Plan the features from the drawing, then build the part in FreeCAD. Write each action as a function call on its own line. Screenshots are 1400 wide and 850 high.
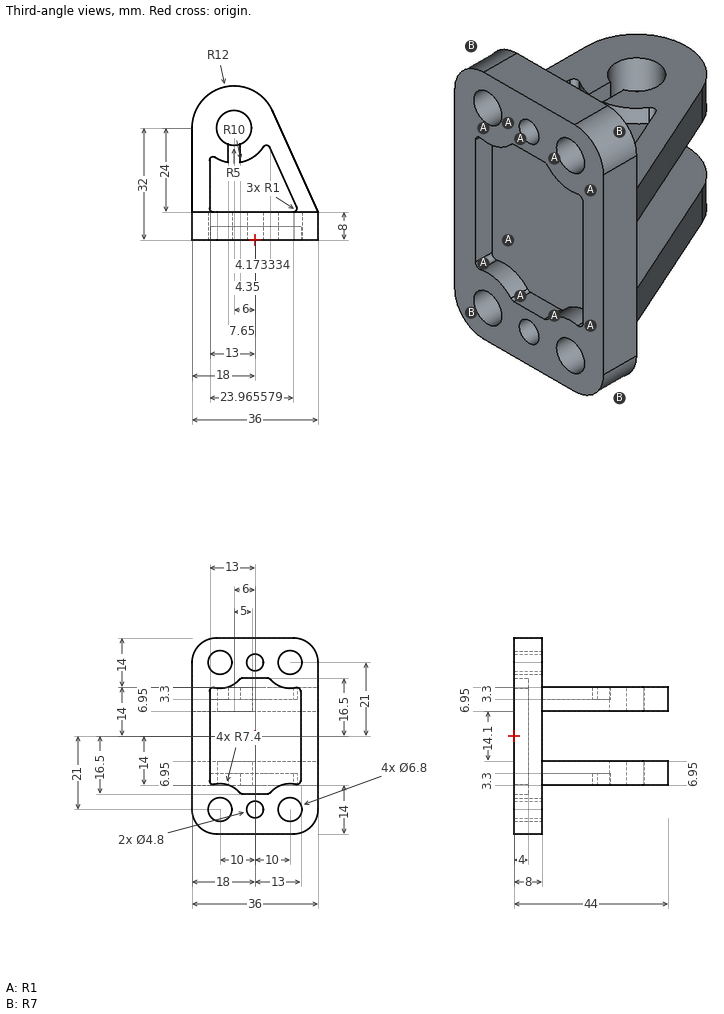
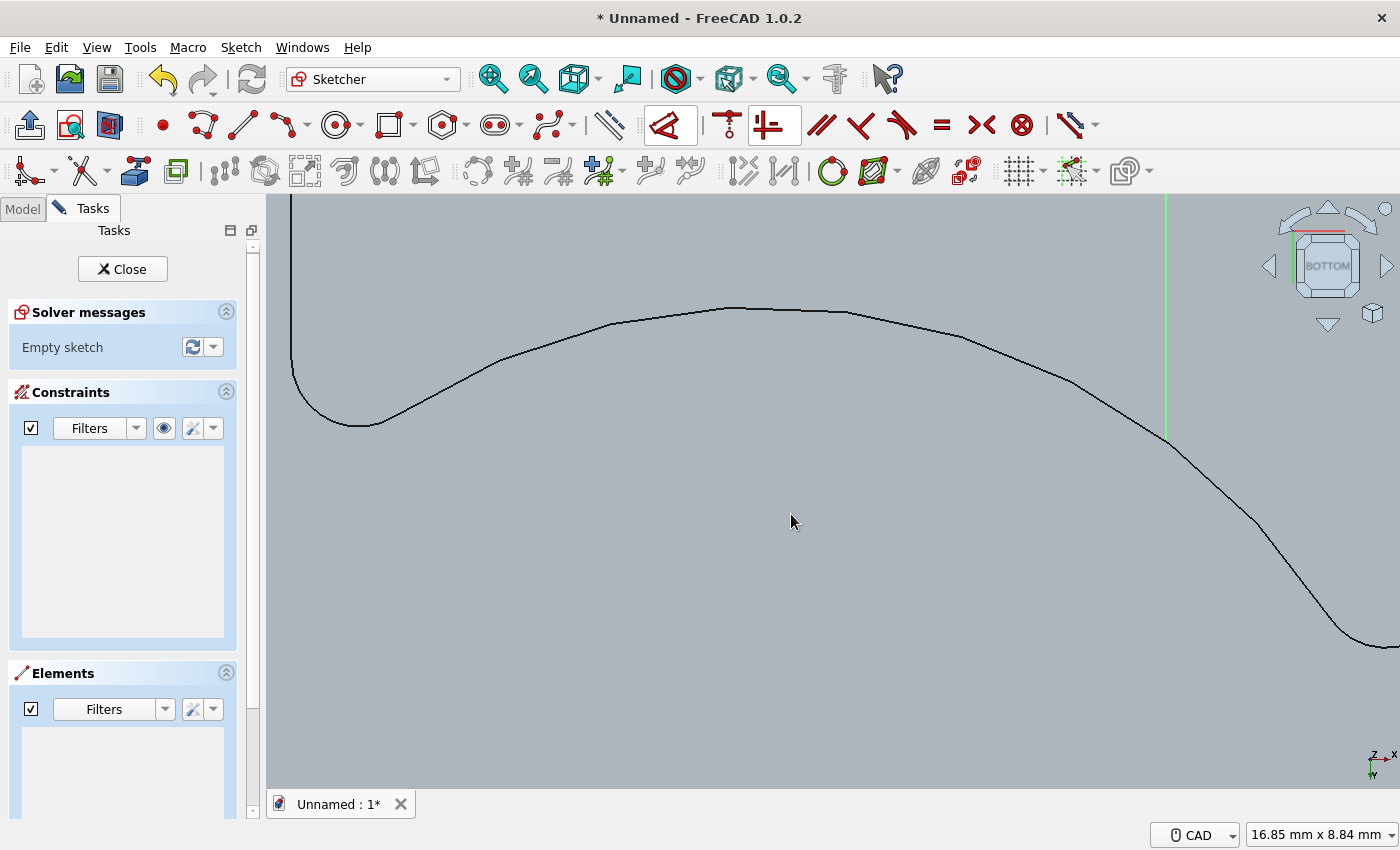
click(244, 126)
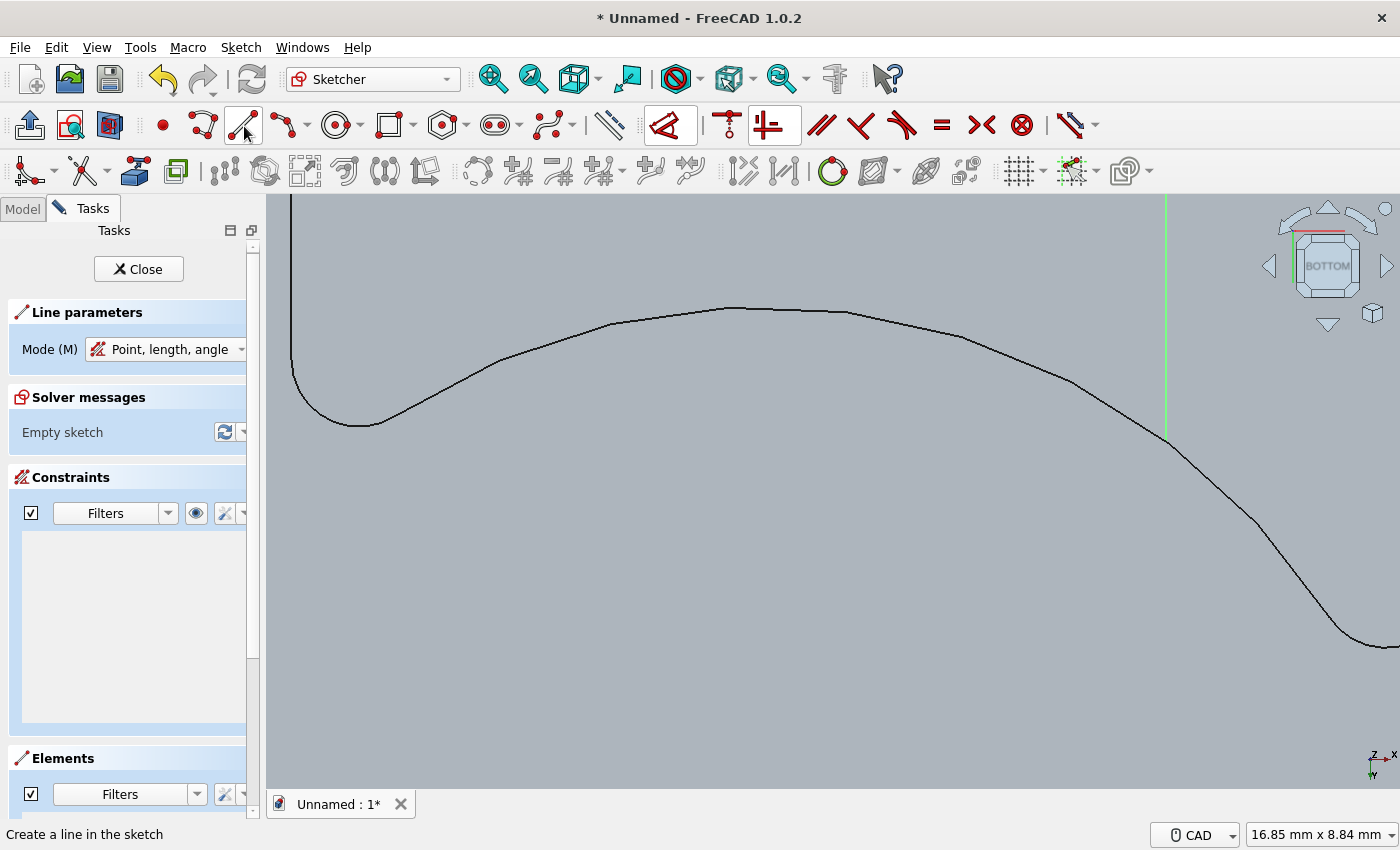
click(652, 316)
click(652, 662)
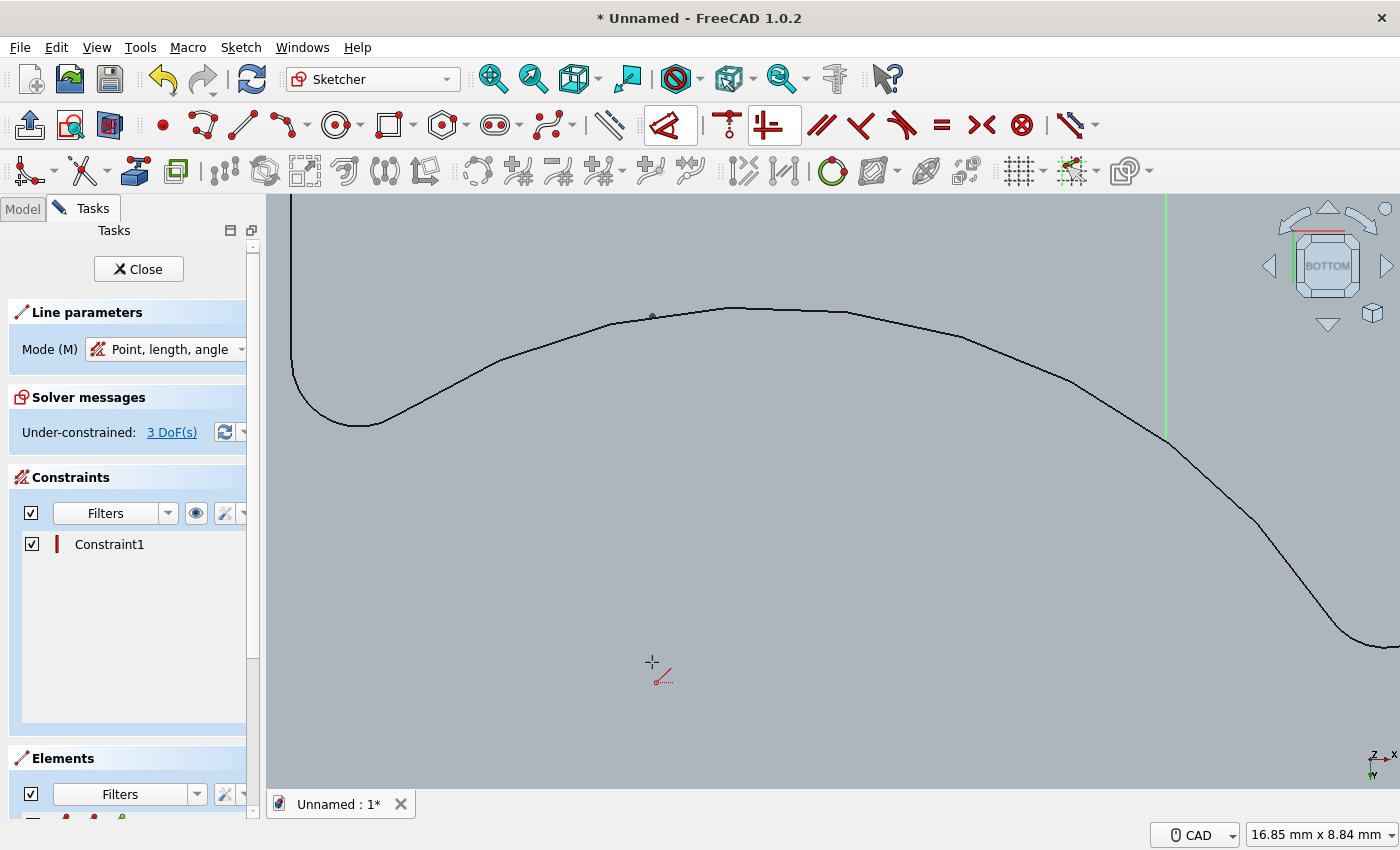
click(874, 662)
click(874, 316)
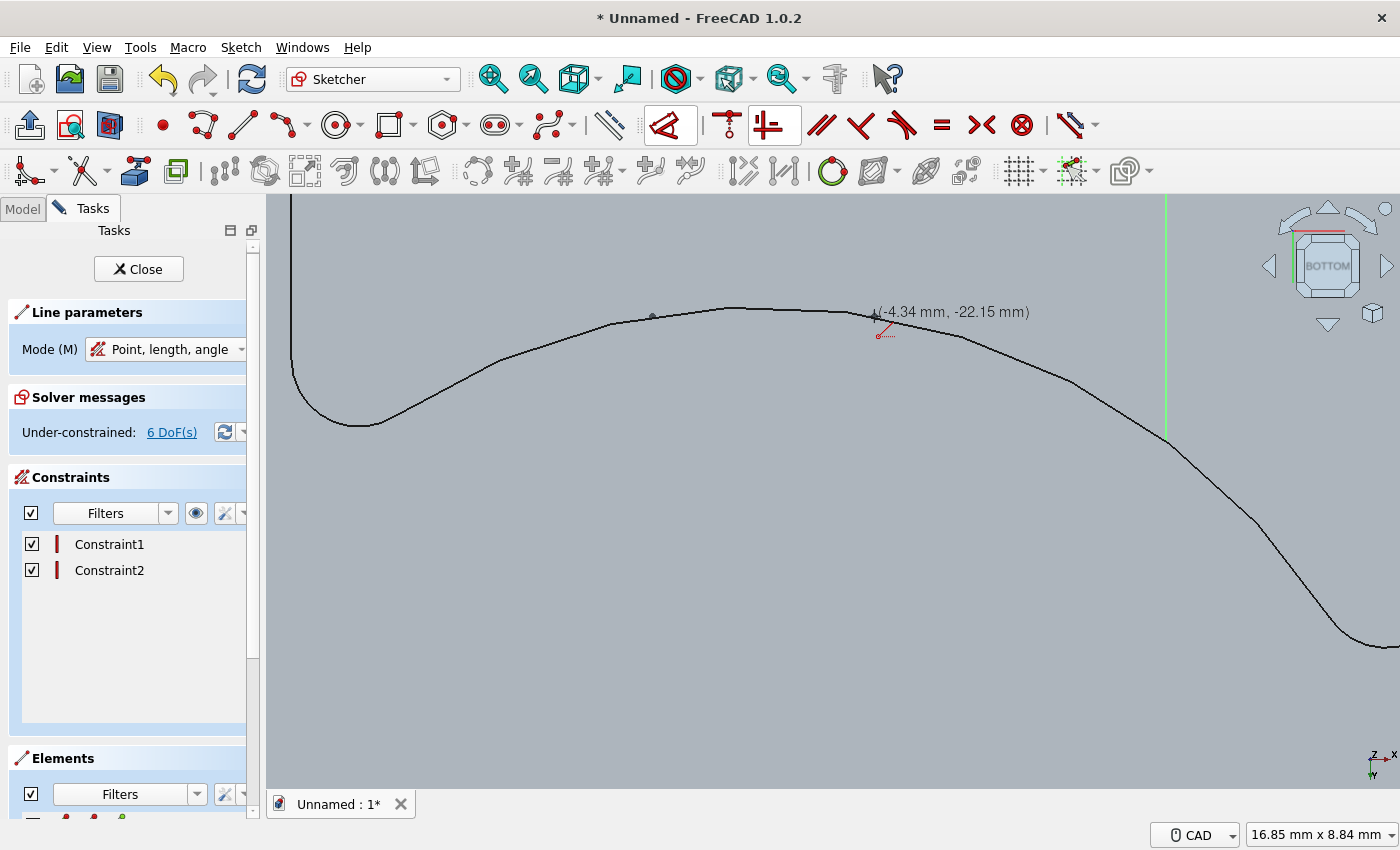
key(g)
key(3)
key(a)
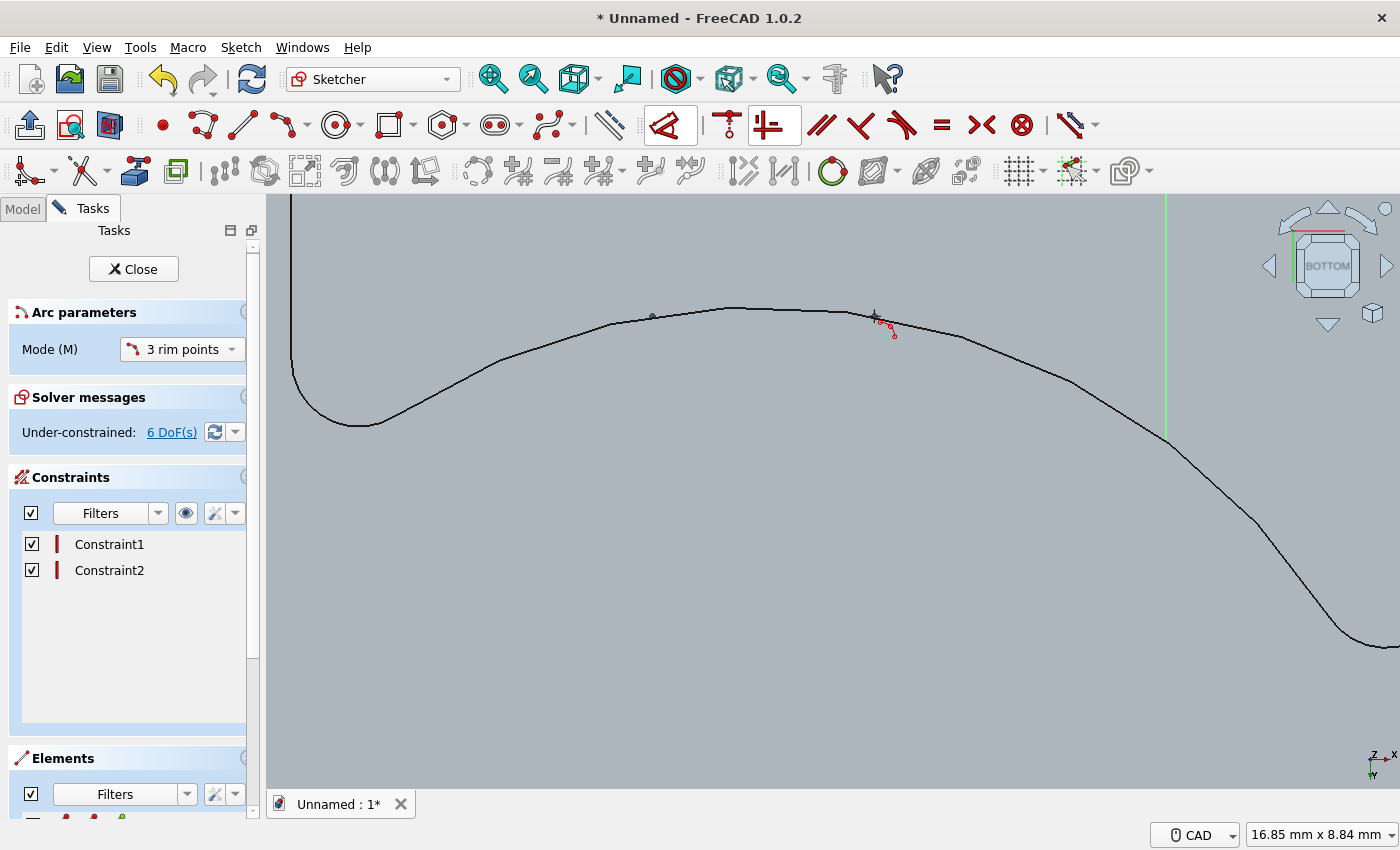
click(652, 663)
click(874, 663)
click(763, 643)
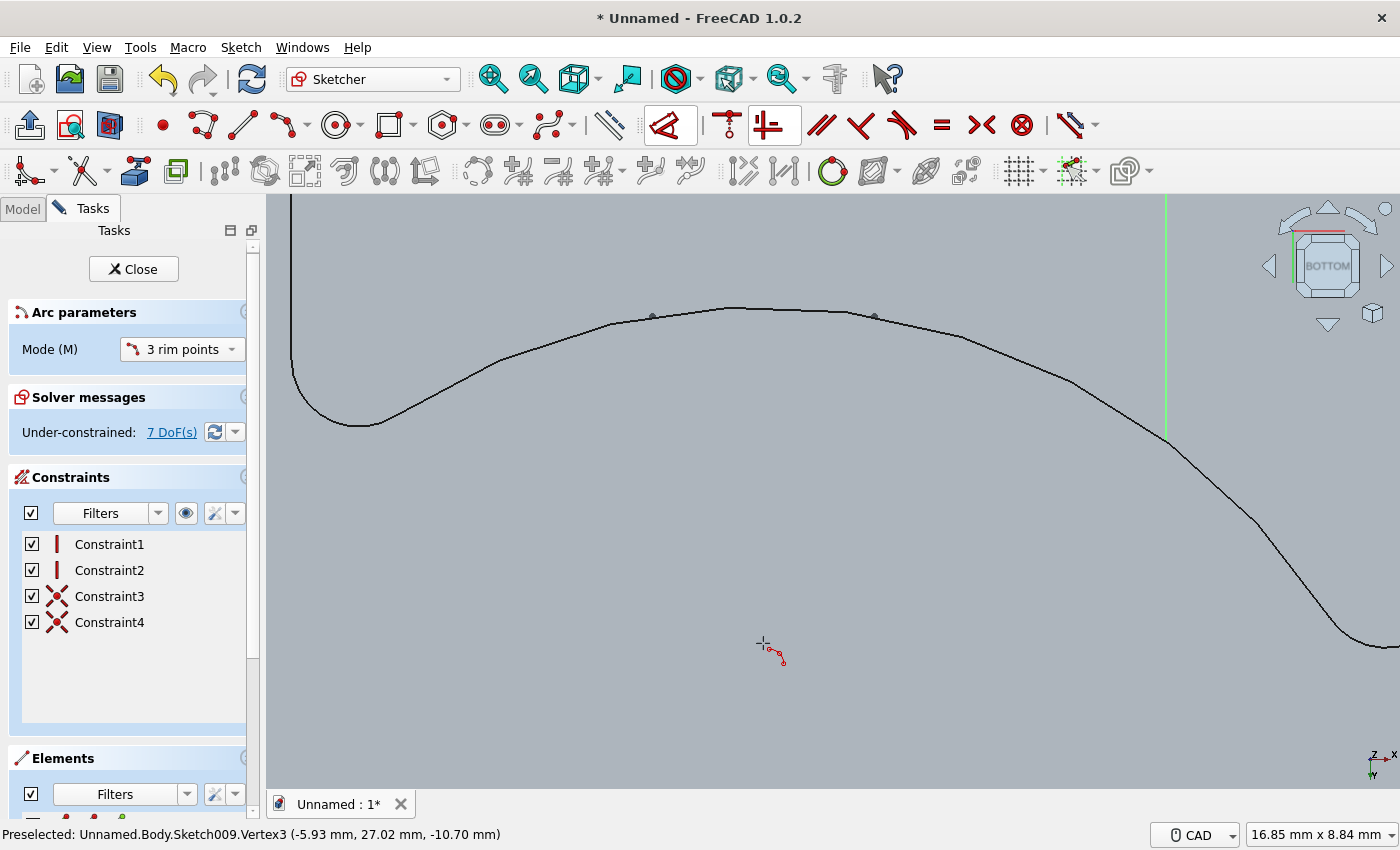
click(874, 317)
click(652, 317)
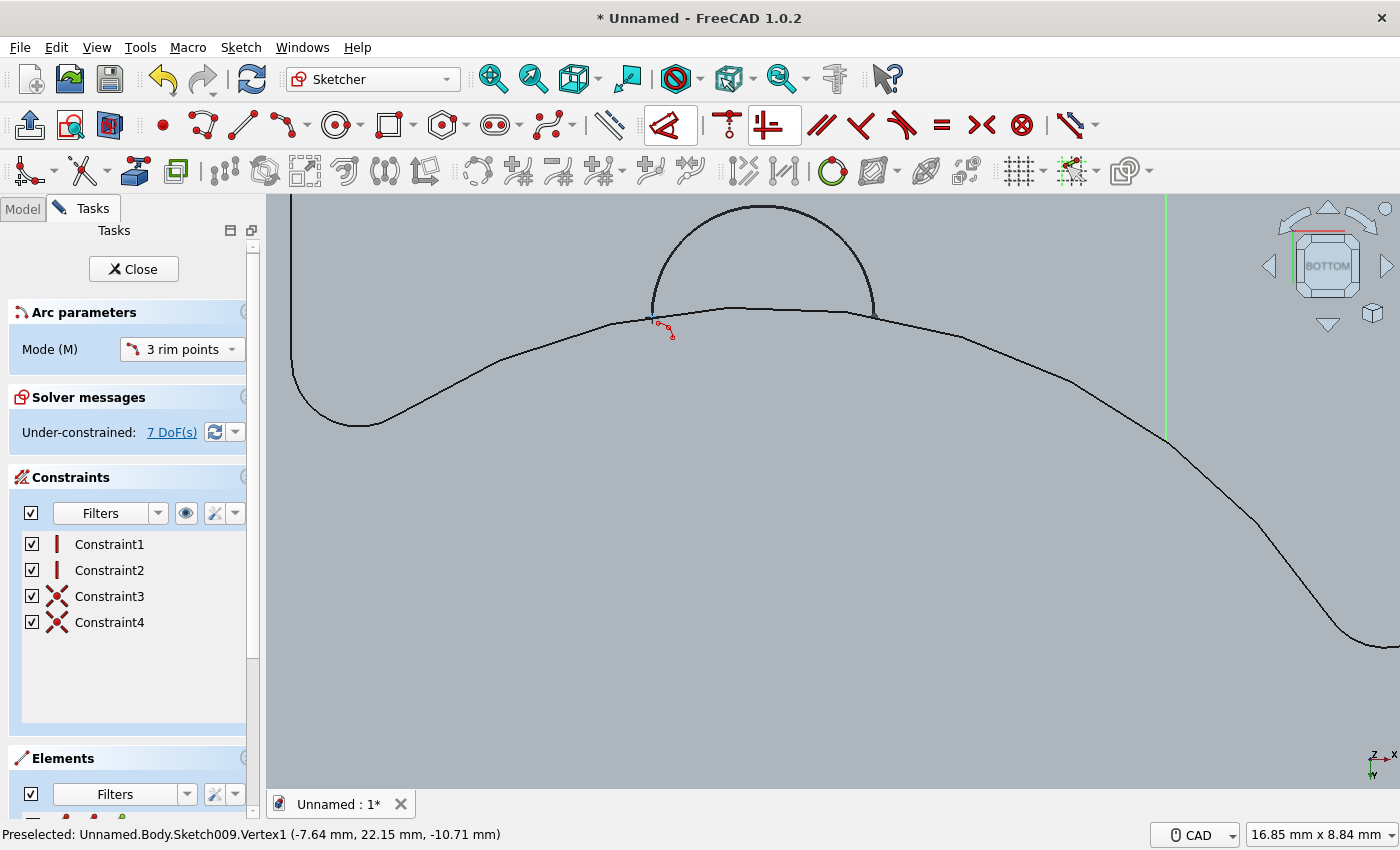
scroll(763, 307, up, 3)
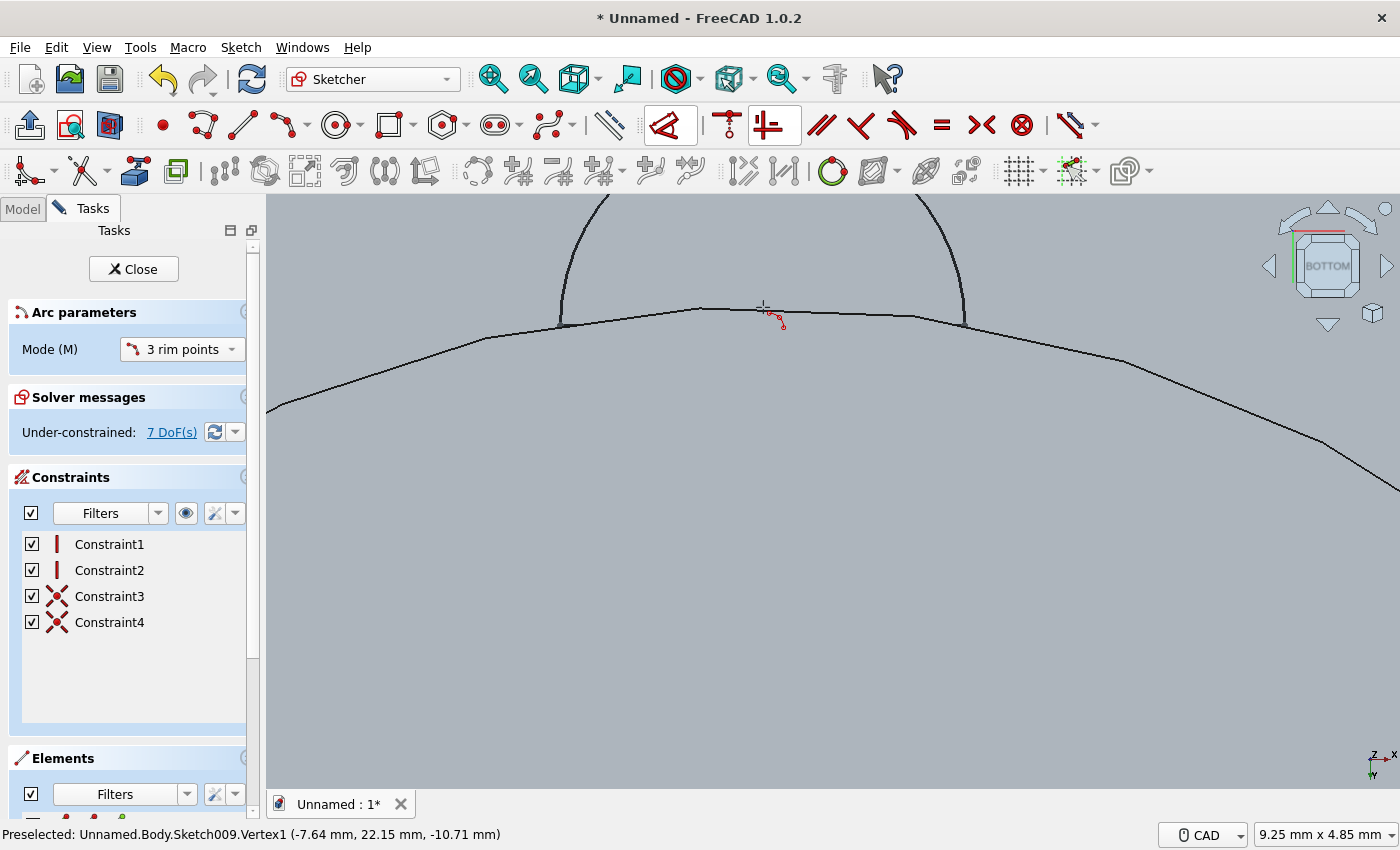
click(762, 307)
key(Escape)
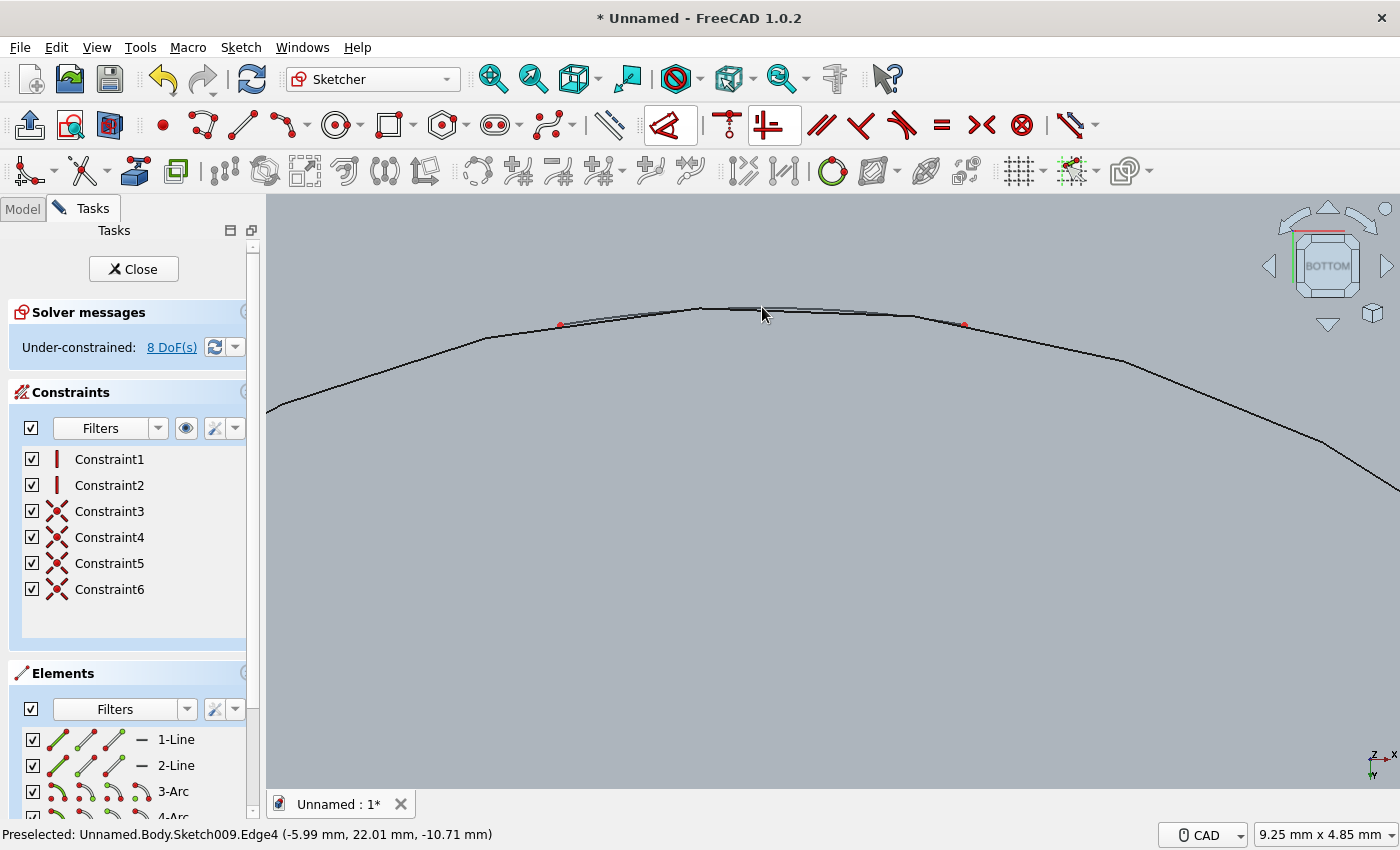
scroll(768, 322, down, 3)